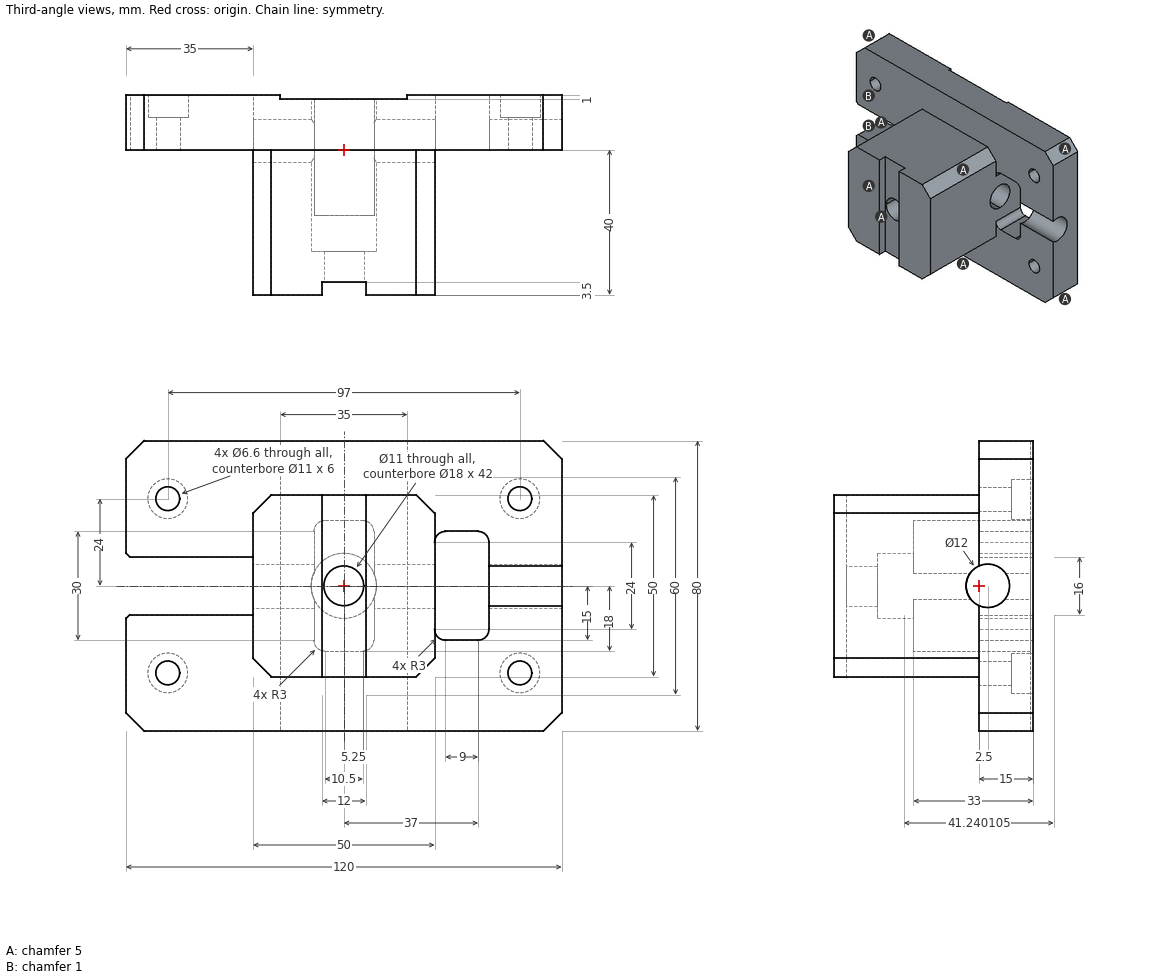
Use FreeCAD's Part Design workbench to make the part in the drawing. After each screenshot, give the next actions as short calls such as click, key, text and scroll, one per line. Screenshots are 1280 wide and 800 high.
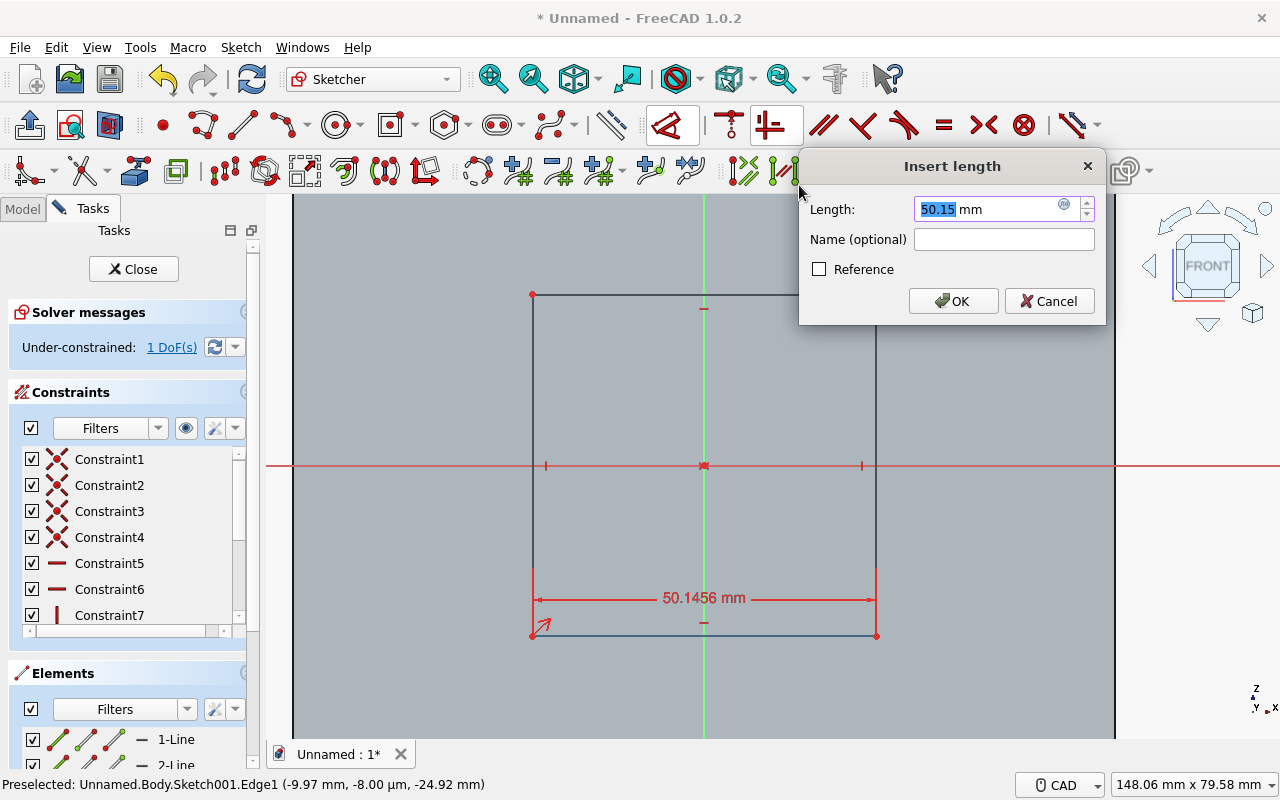
text(50)
key(Return)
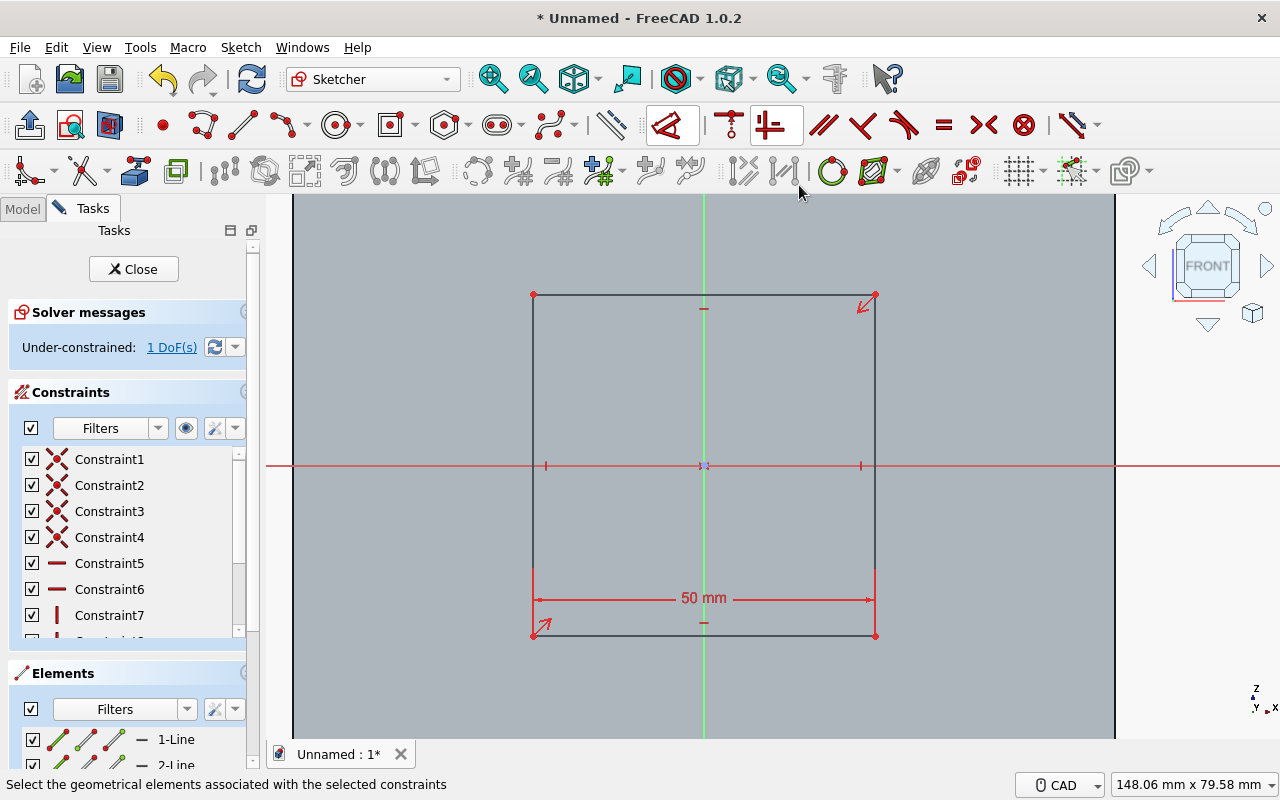
click(876, 534)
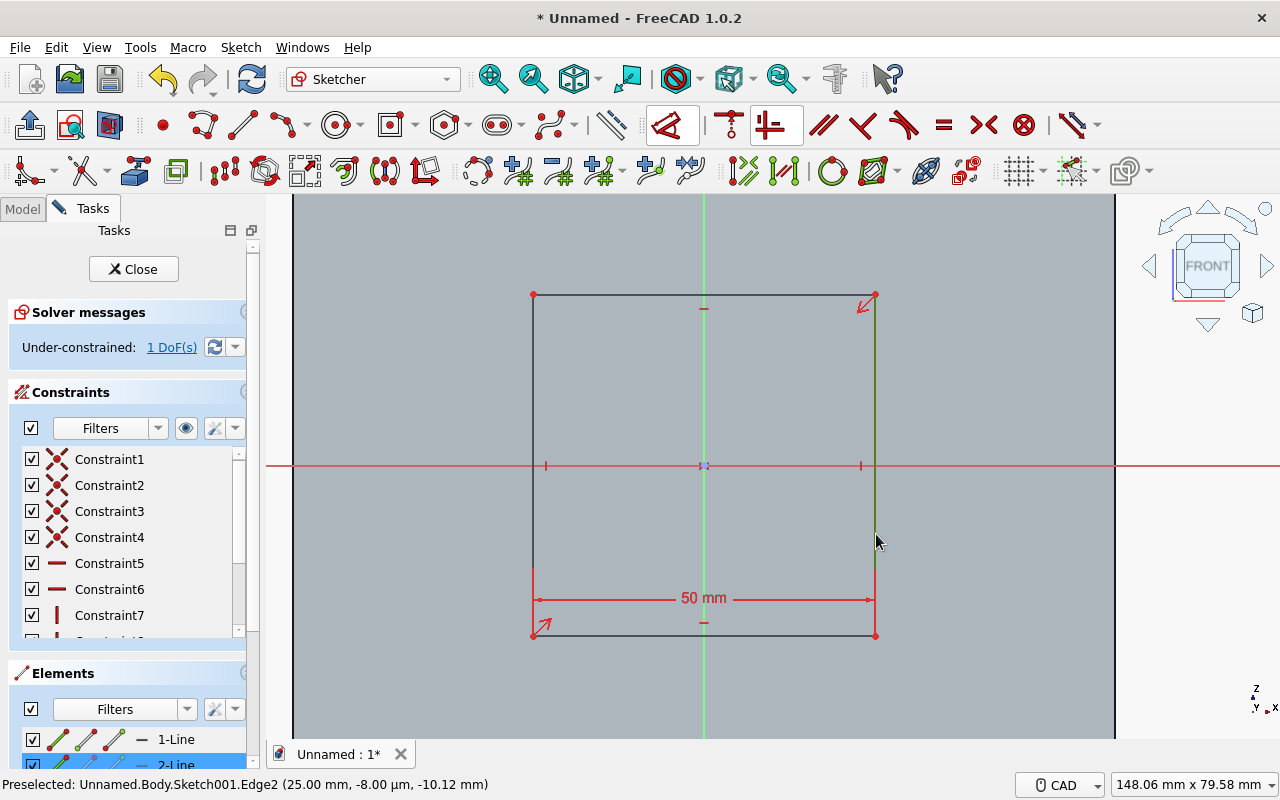
key(i)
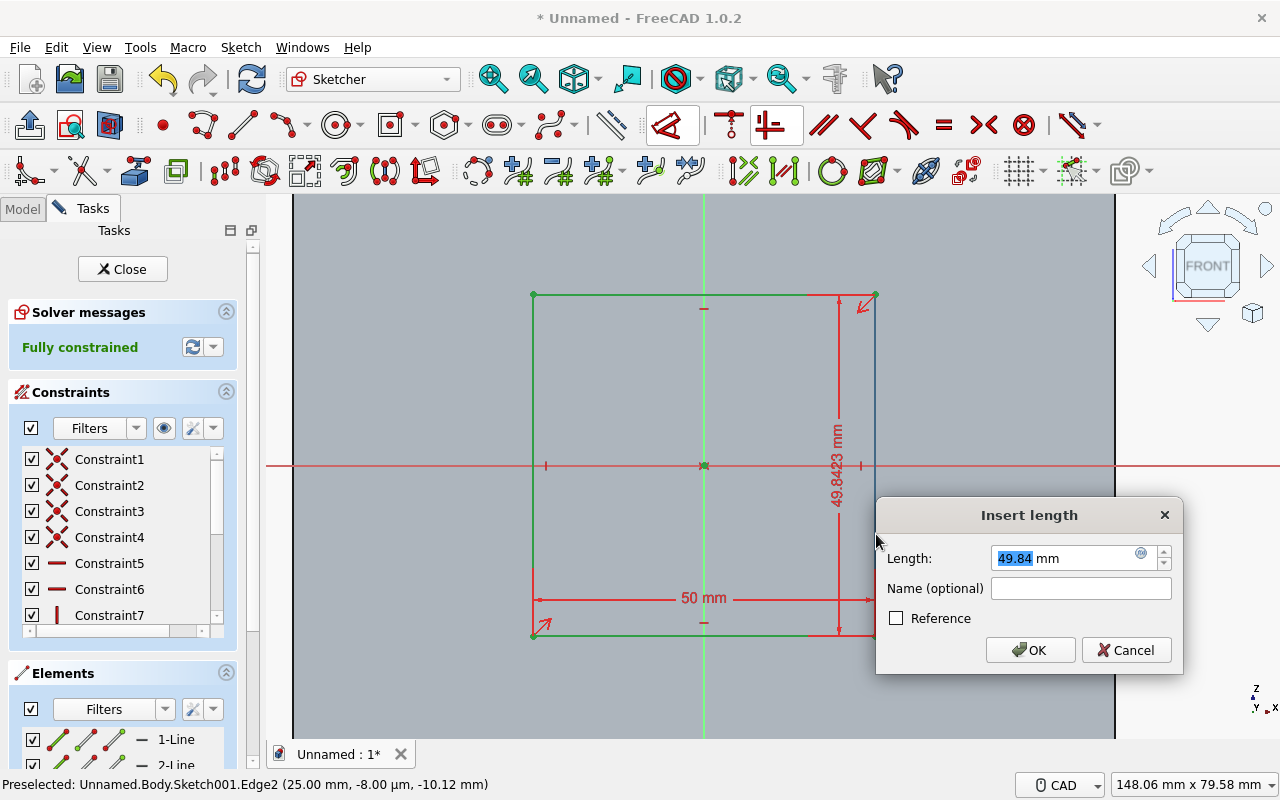
text(50)
key(Return)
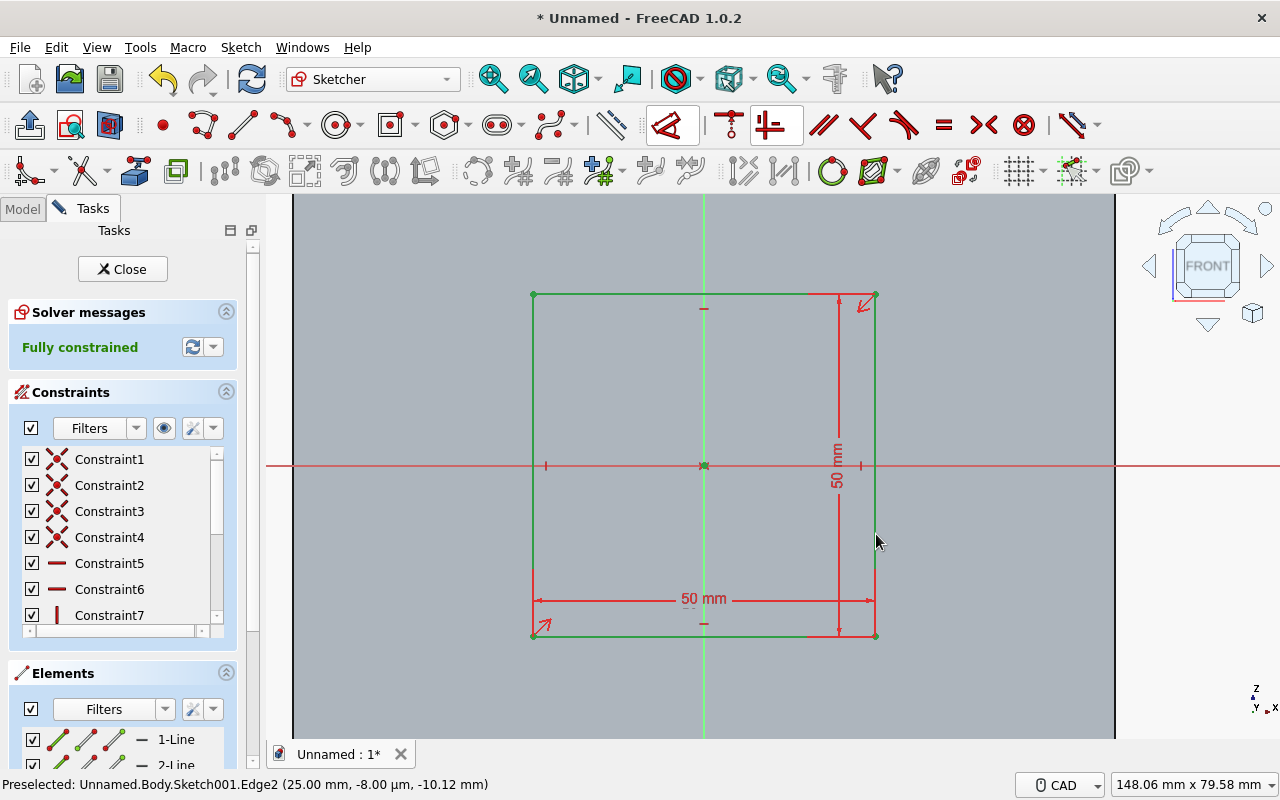
click(123, 269)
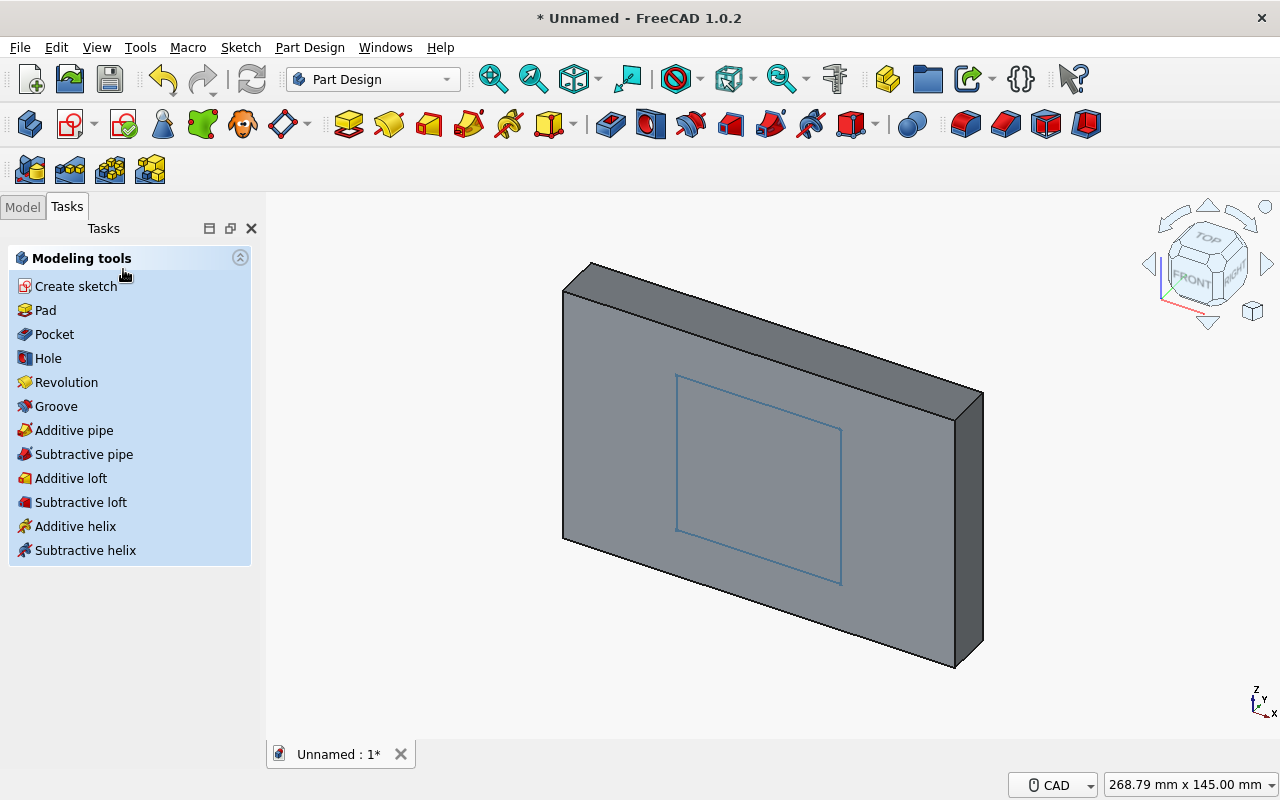
click(350, 124)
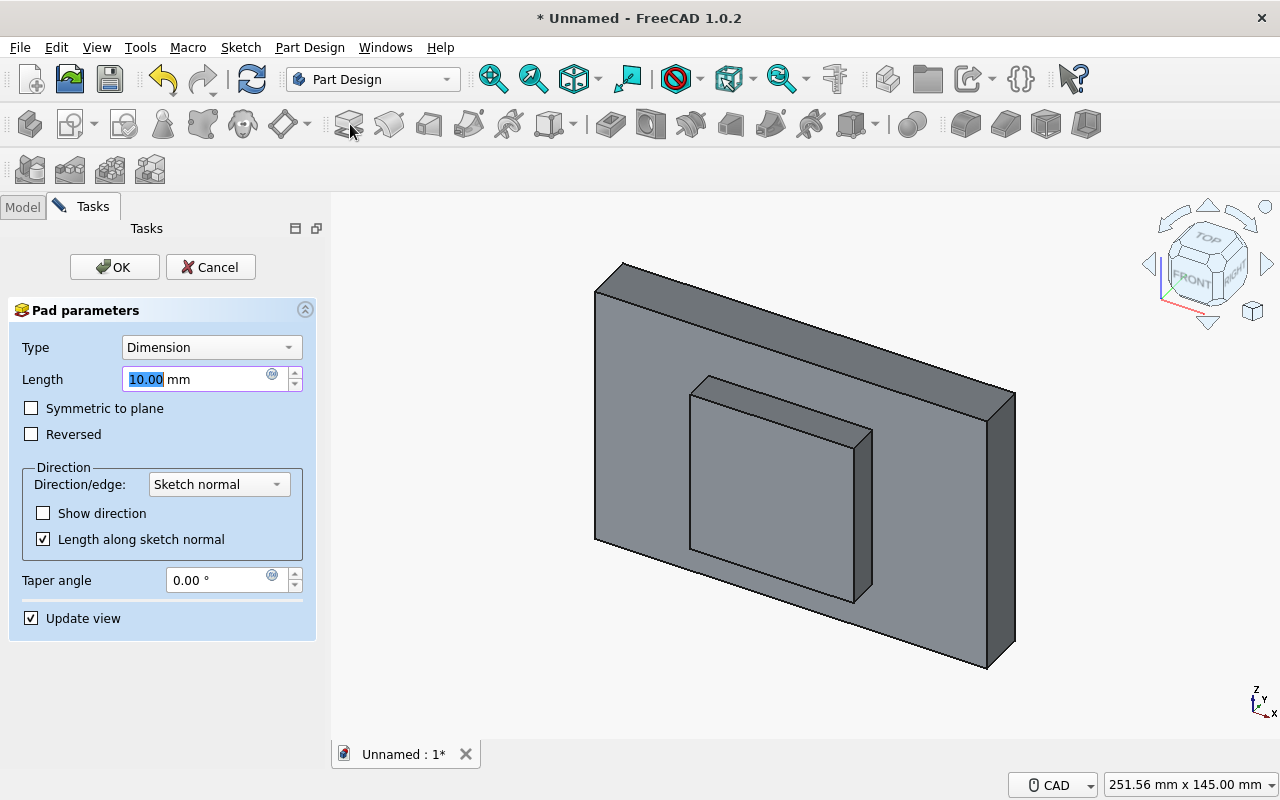
text(40)
key(Tab)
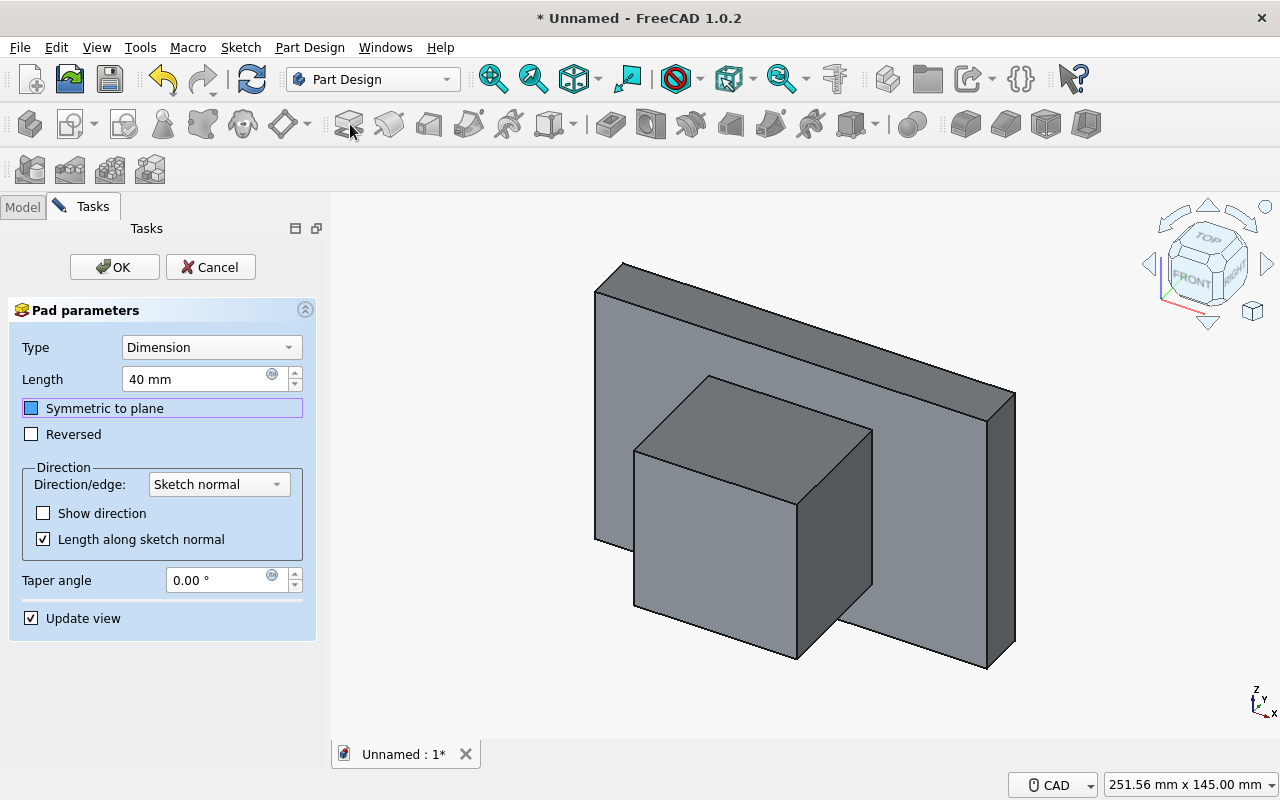
click(115, 267)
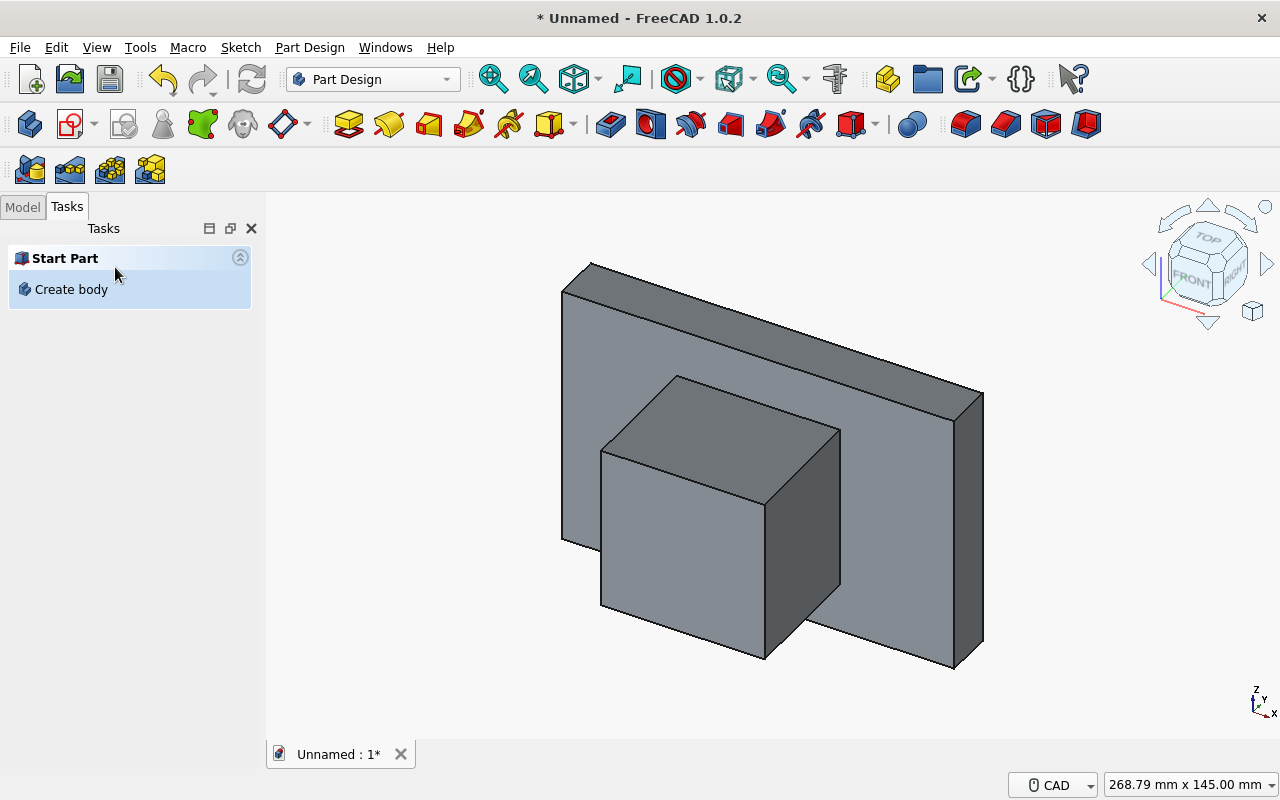
click(494, 80)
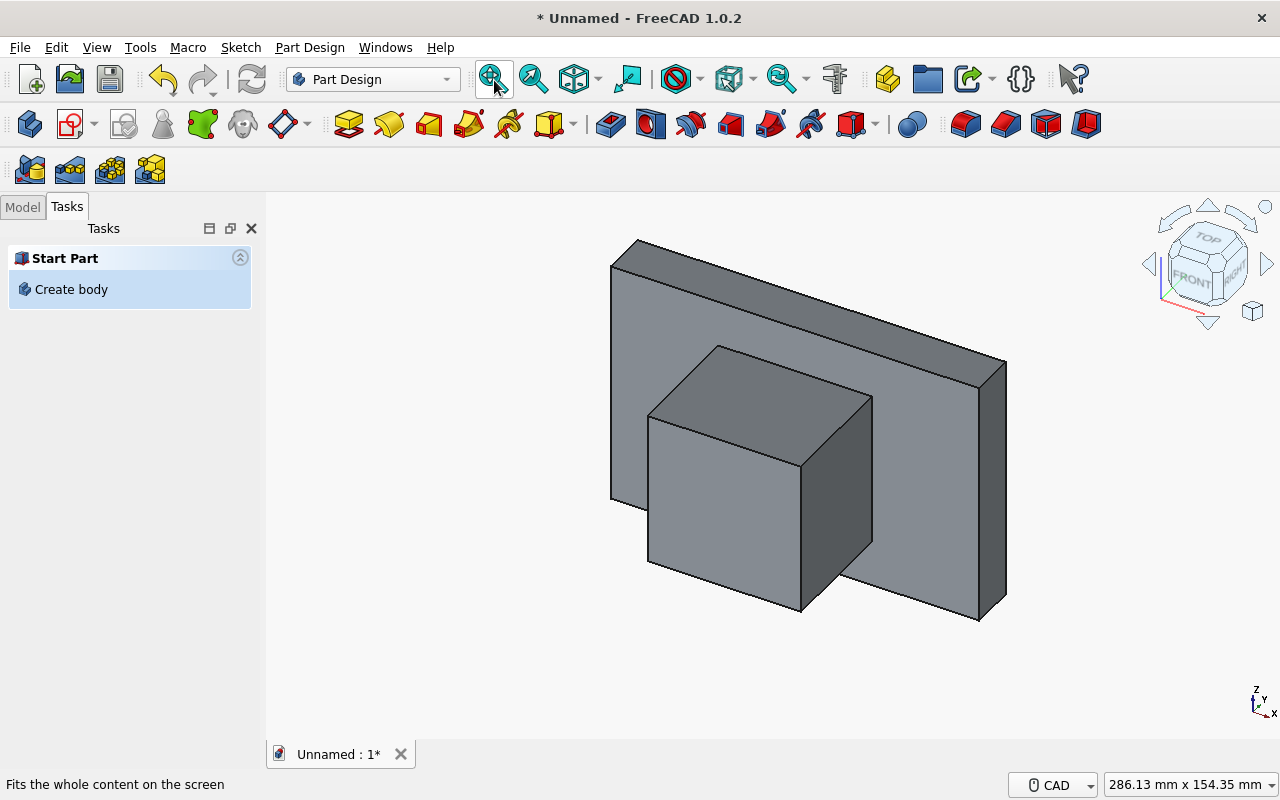
key(4)